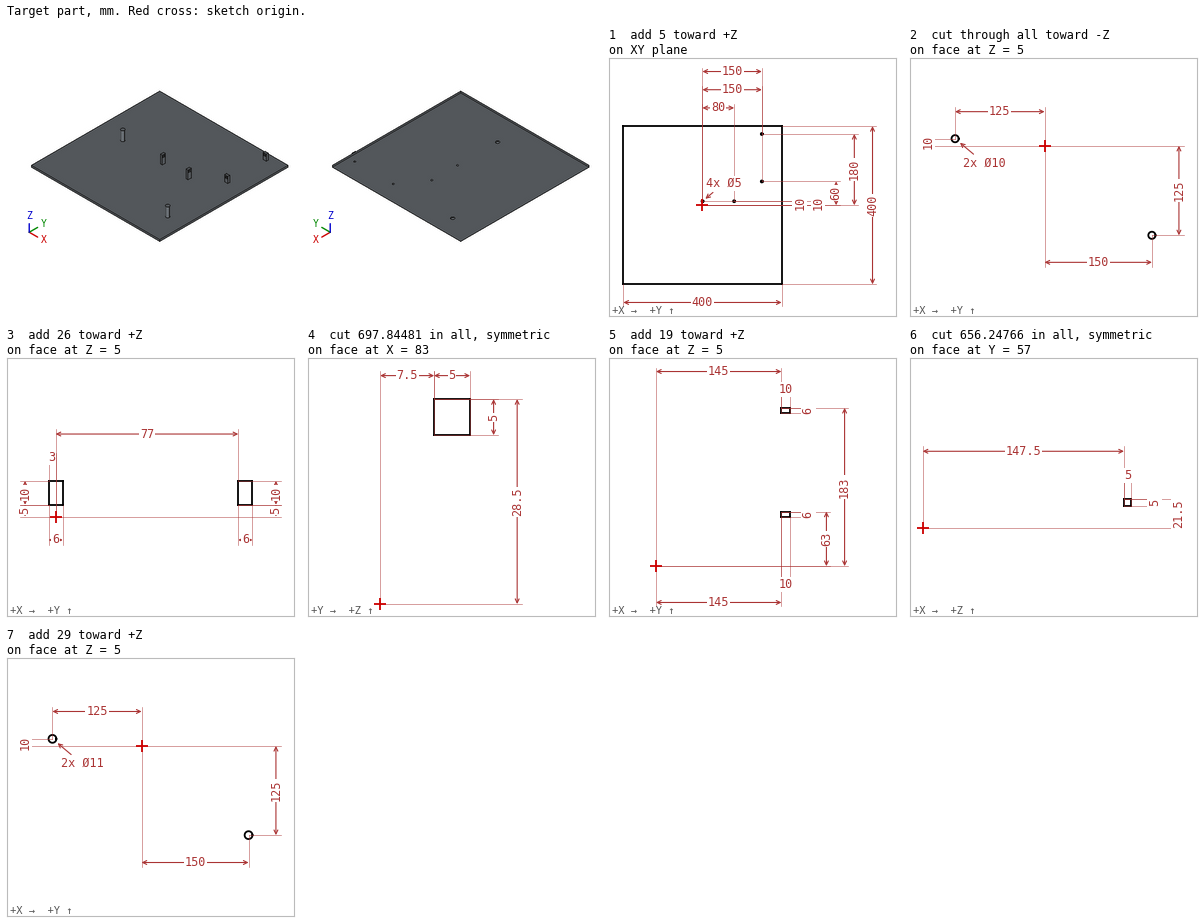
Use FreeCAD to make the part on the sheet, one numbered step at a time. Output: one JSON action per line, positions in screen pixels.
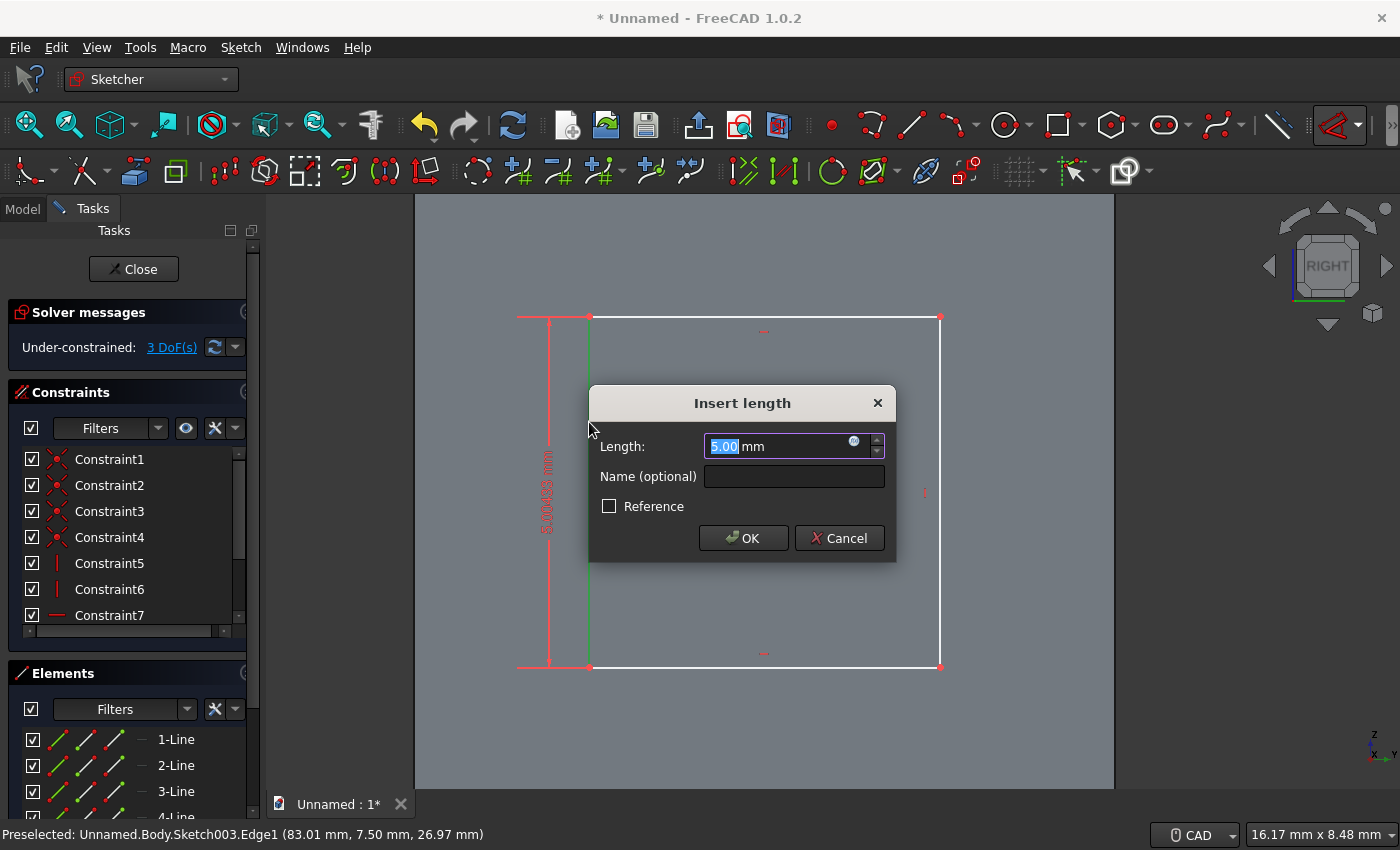
{"action": "type", "text": "5"}
{"action": "key", "text": "Return"}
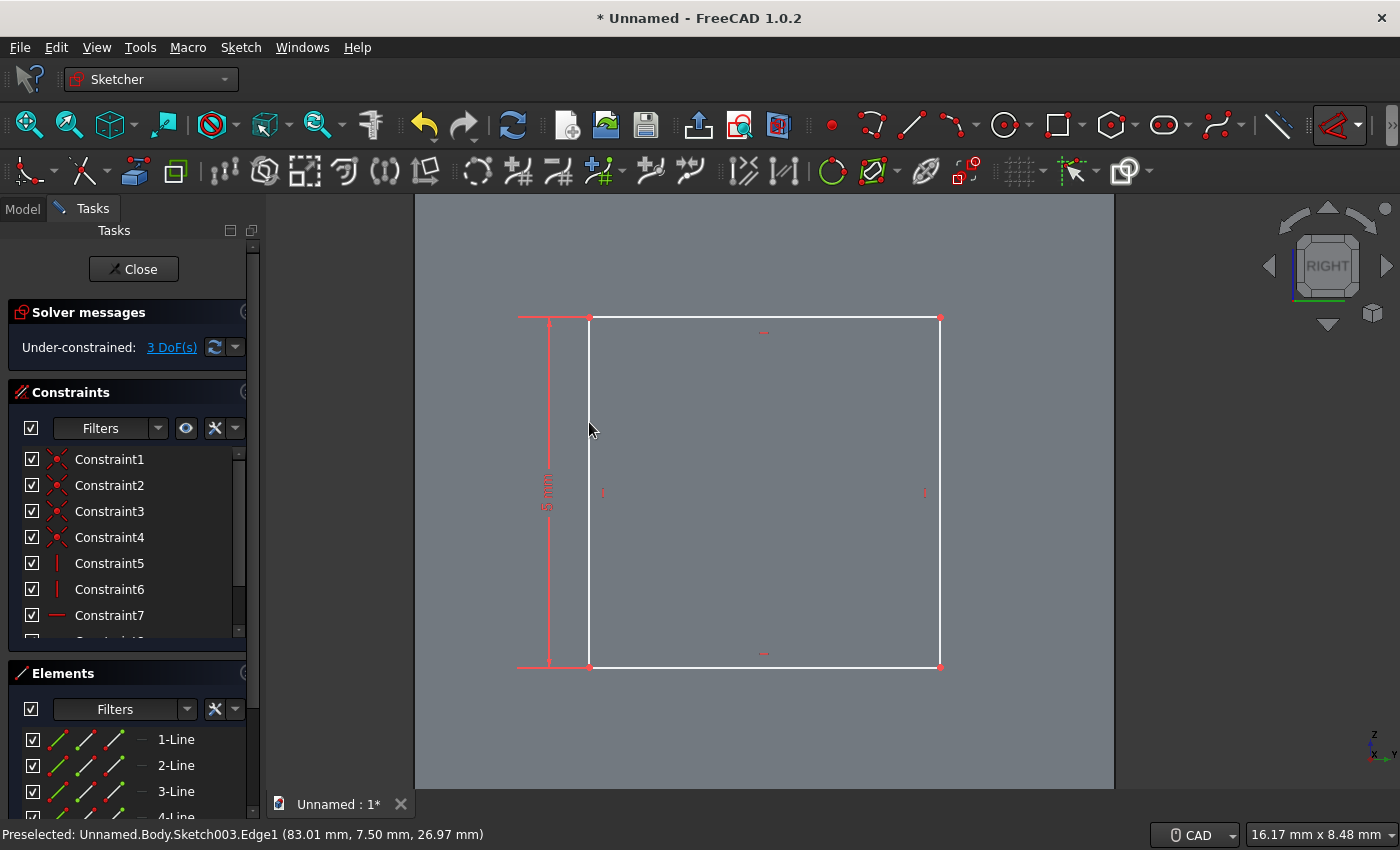
{"action": "left_click", "coordinate": [694, 668]}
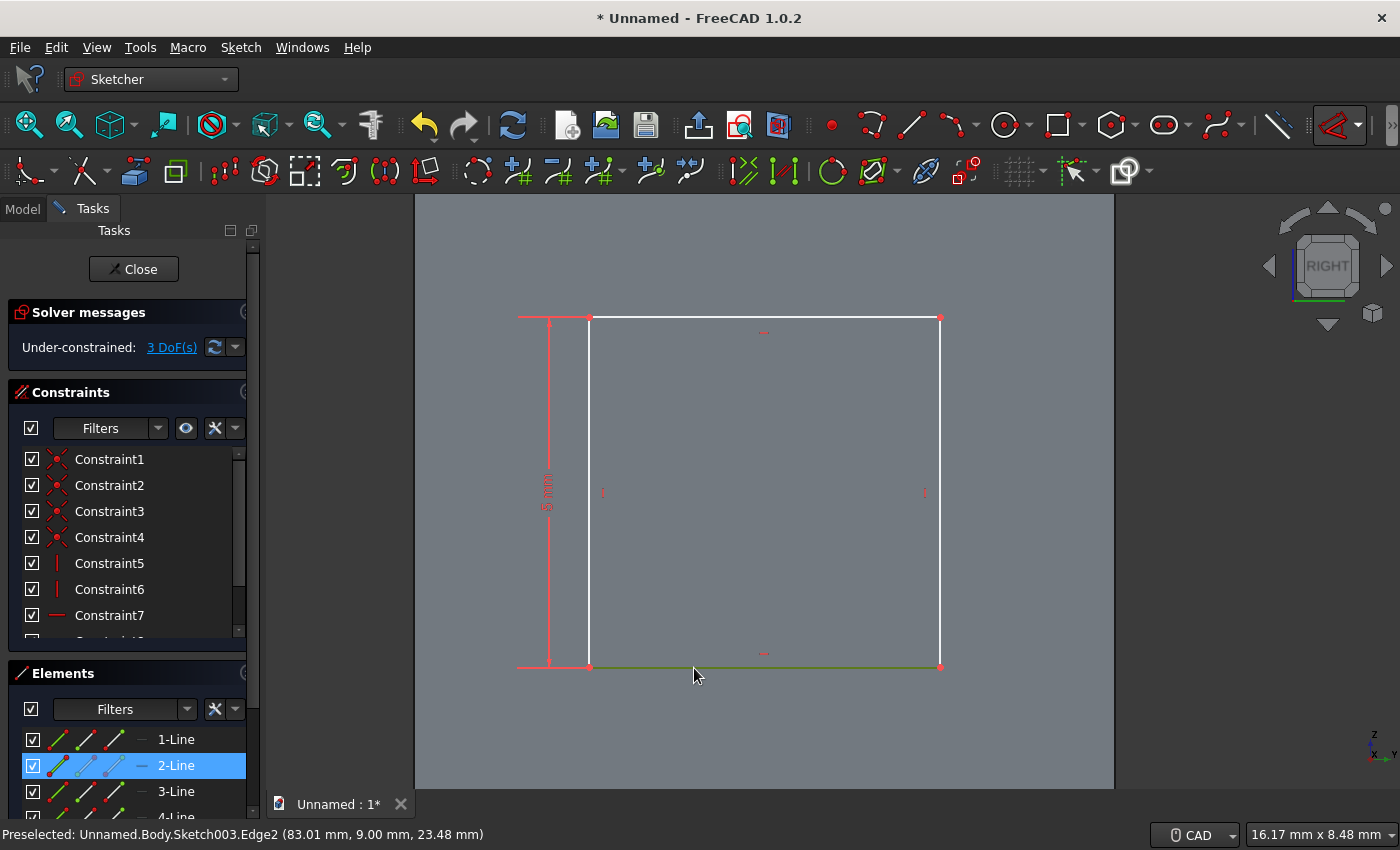
{"action": "key", "text": "l"}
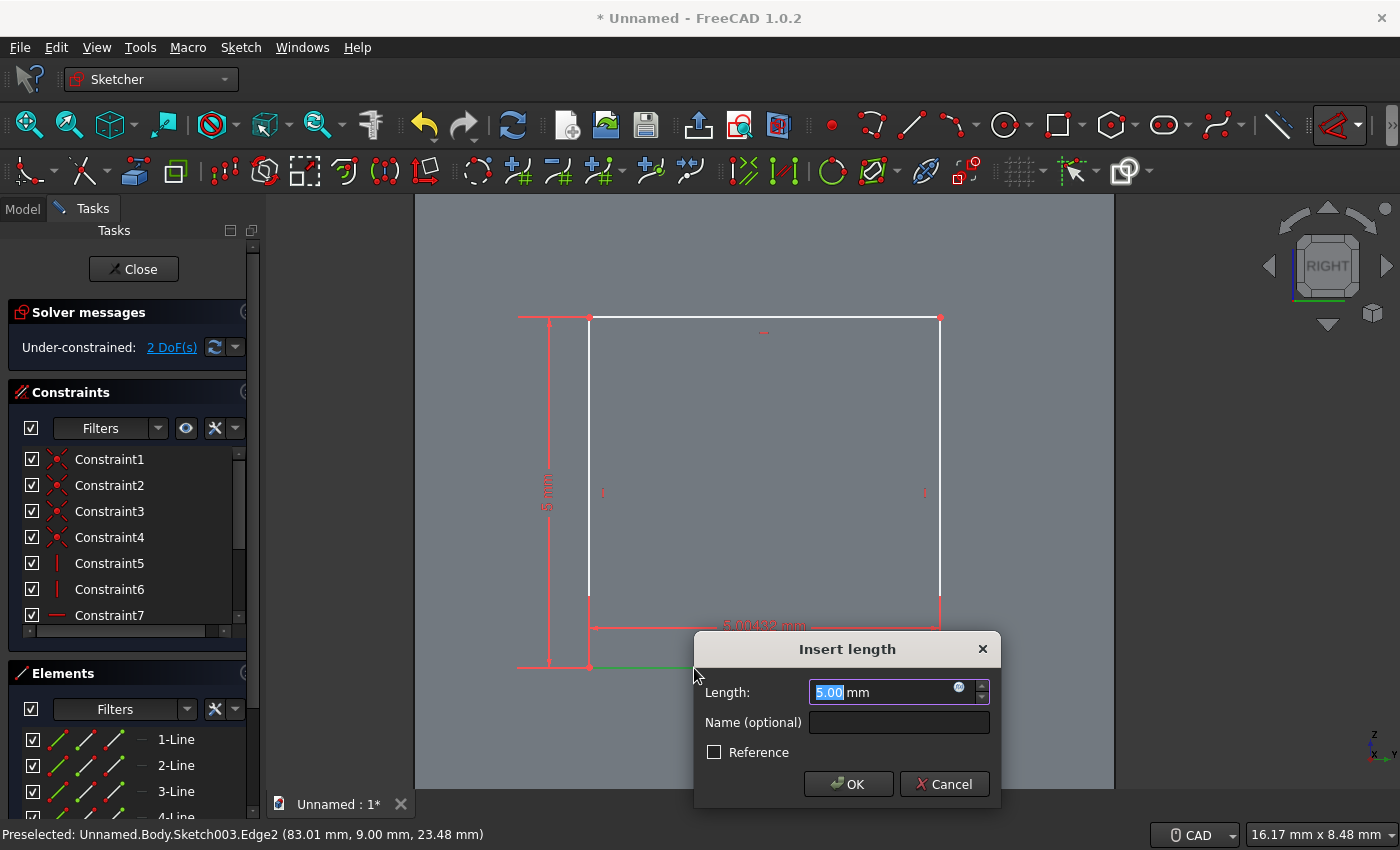
{"action": "type", "text": "5"}
{"action": "key", "text": "Return"}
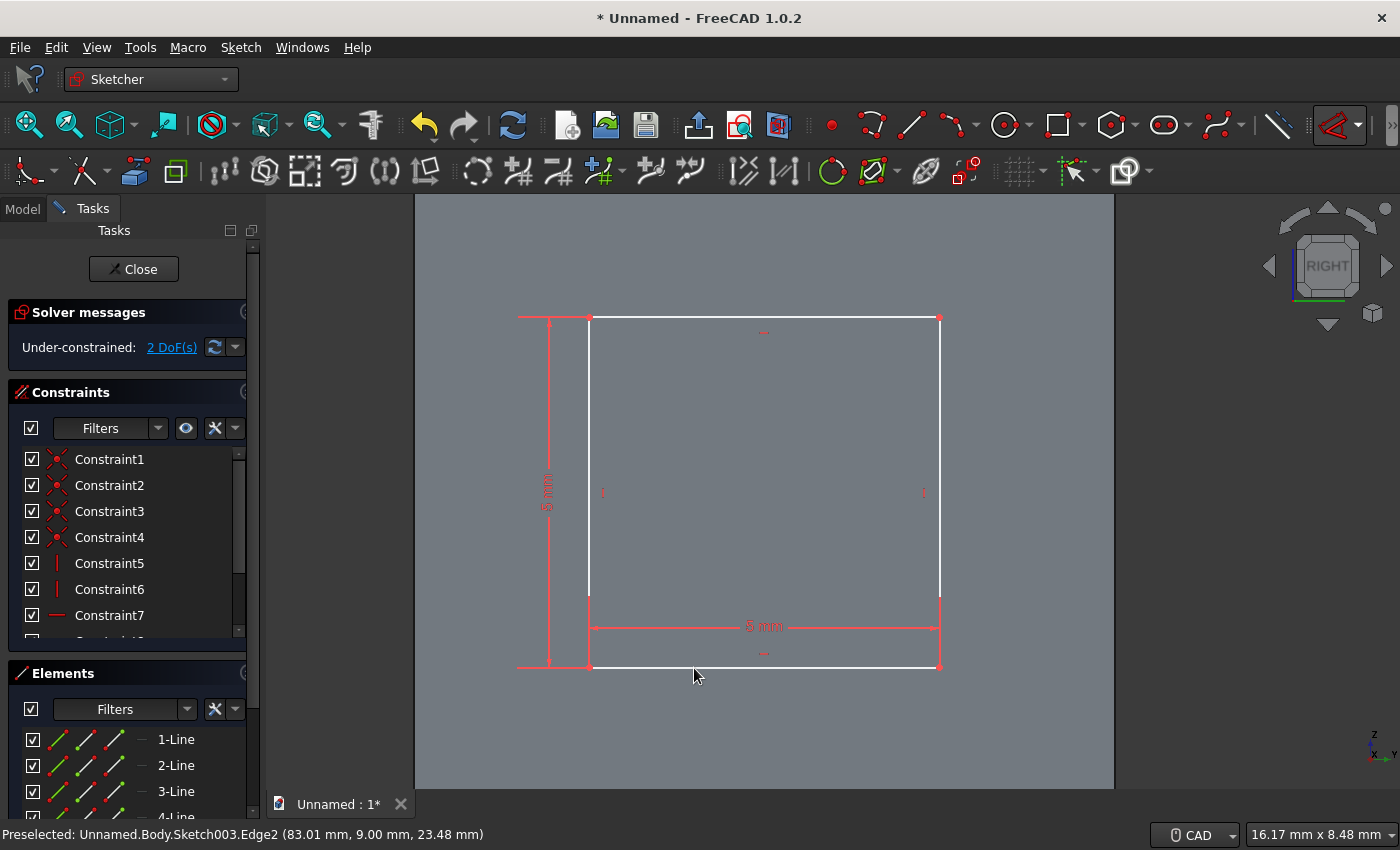
{"action": "left_click", "coordinate": [589, 317]}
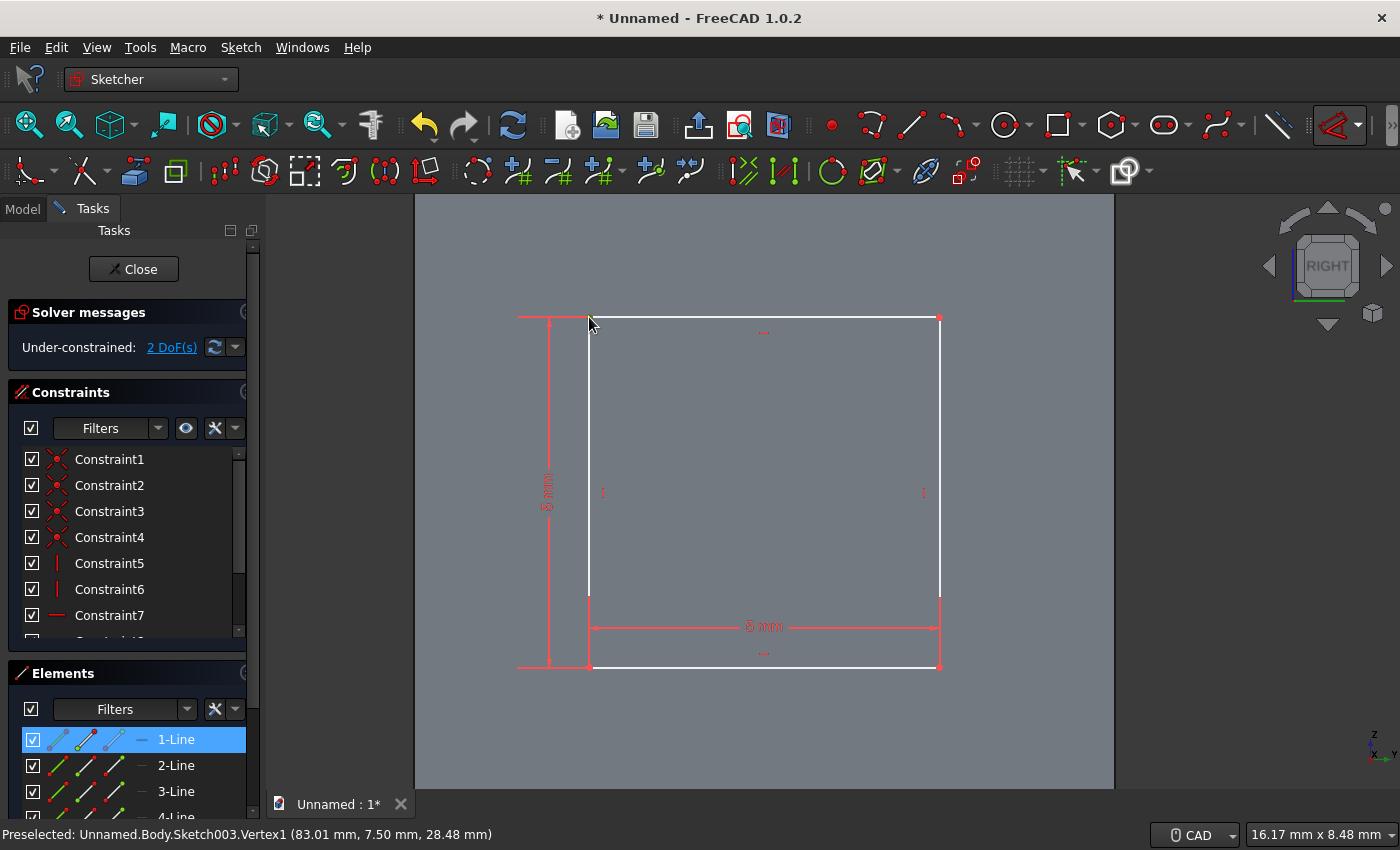
{"action": "key", "text": "l"}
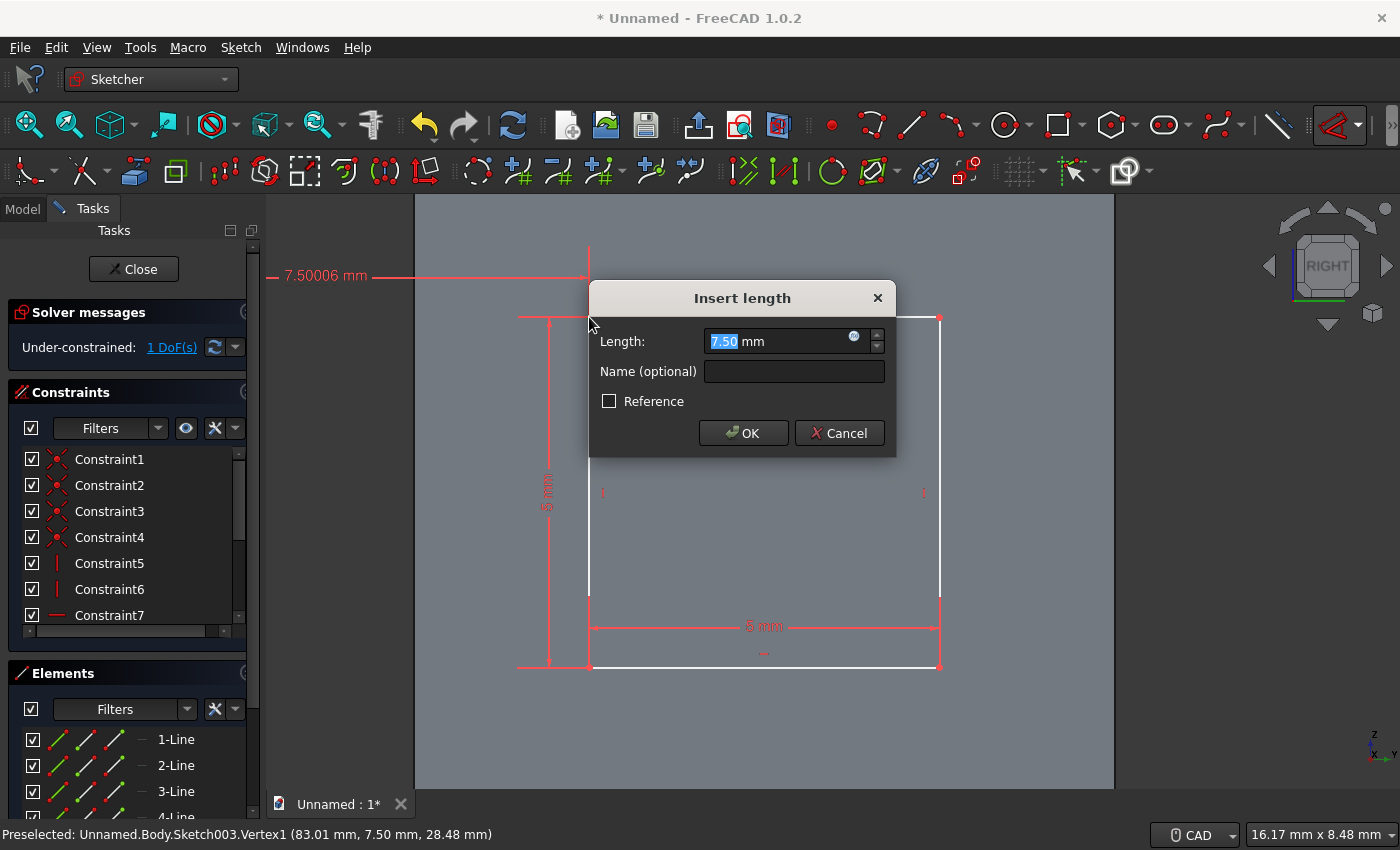
{"action": "type", "text": "7.5"}
{"action": "key", "text": "Return"}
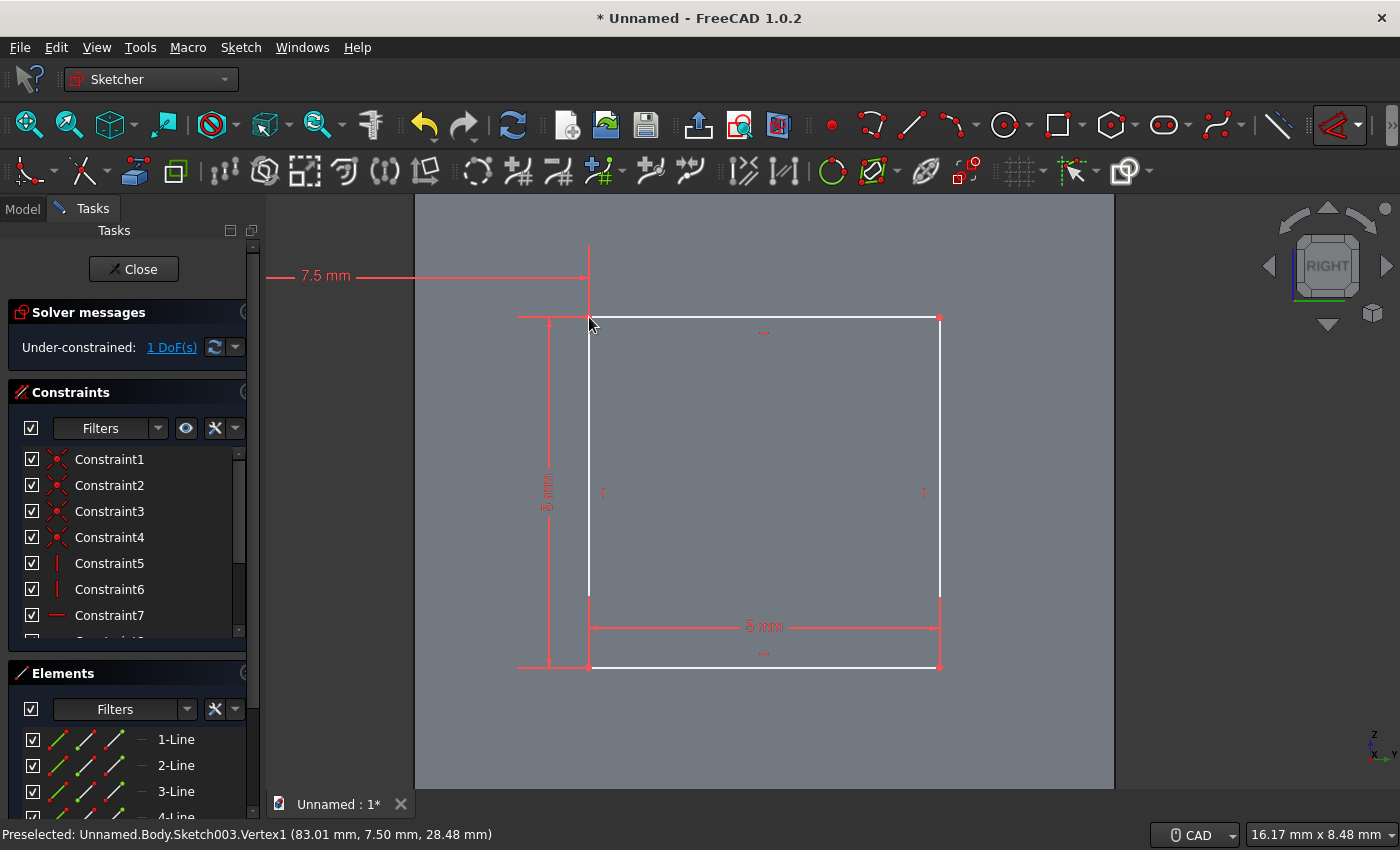
{"action": "left_click", "coordinate": [589, 317]}